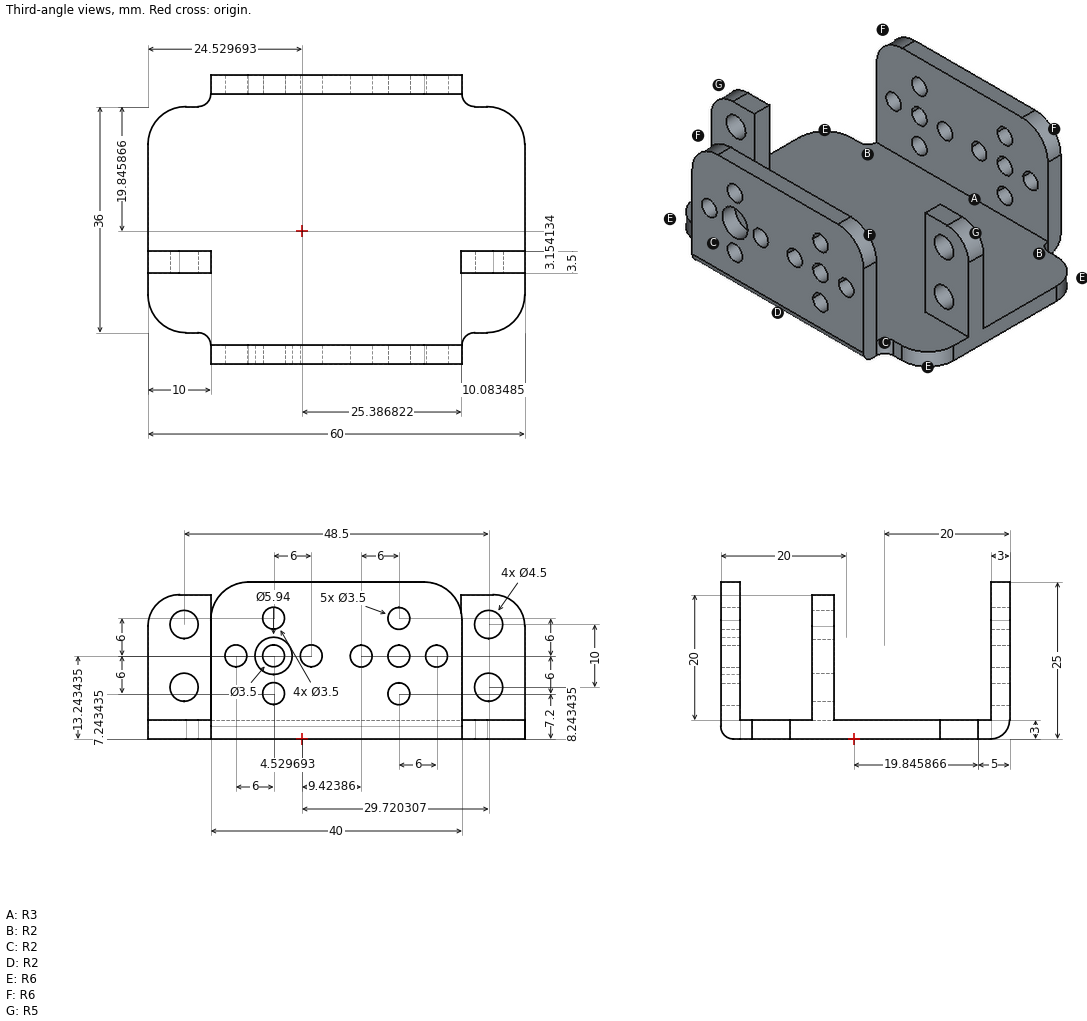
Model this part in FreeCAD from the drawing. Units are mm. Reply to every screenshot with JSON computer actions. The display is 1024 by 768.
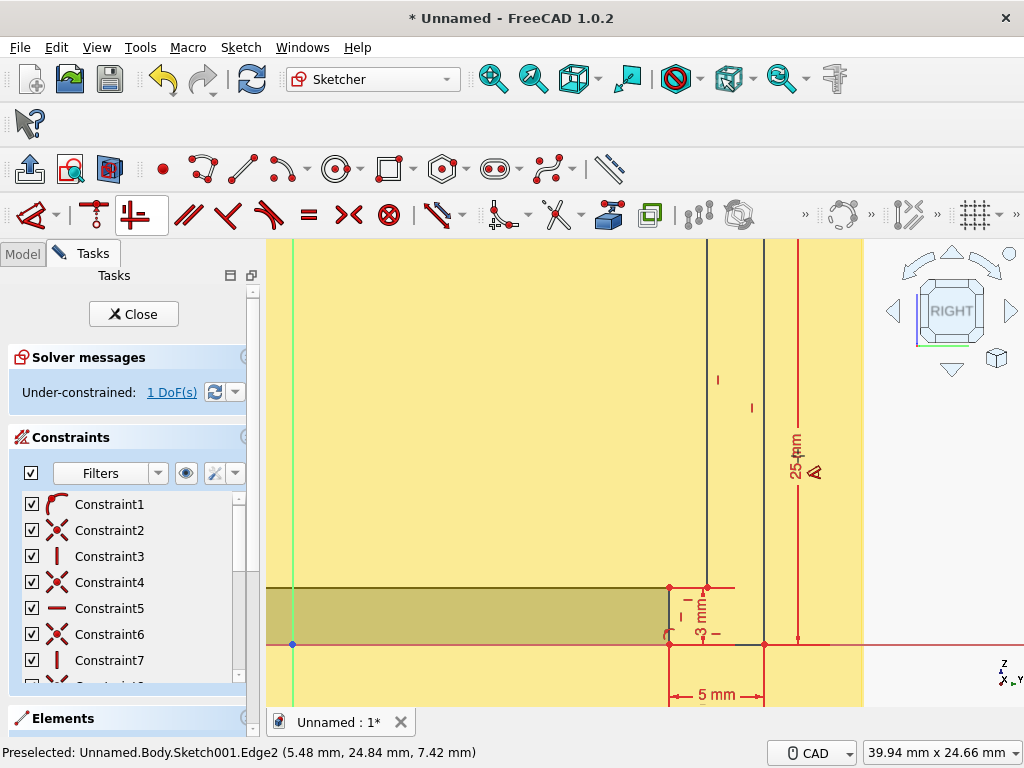
{"action": "left_click", "coordinate": [669, 645]}
{"action": "left_click", "coordinate": [482, 679]}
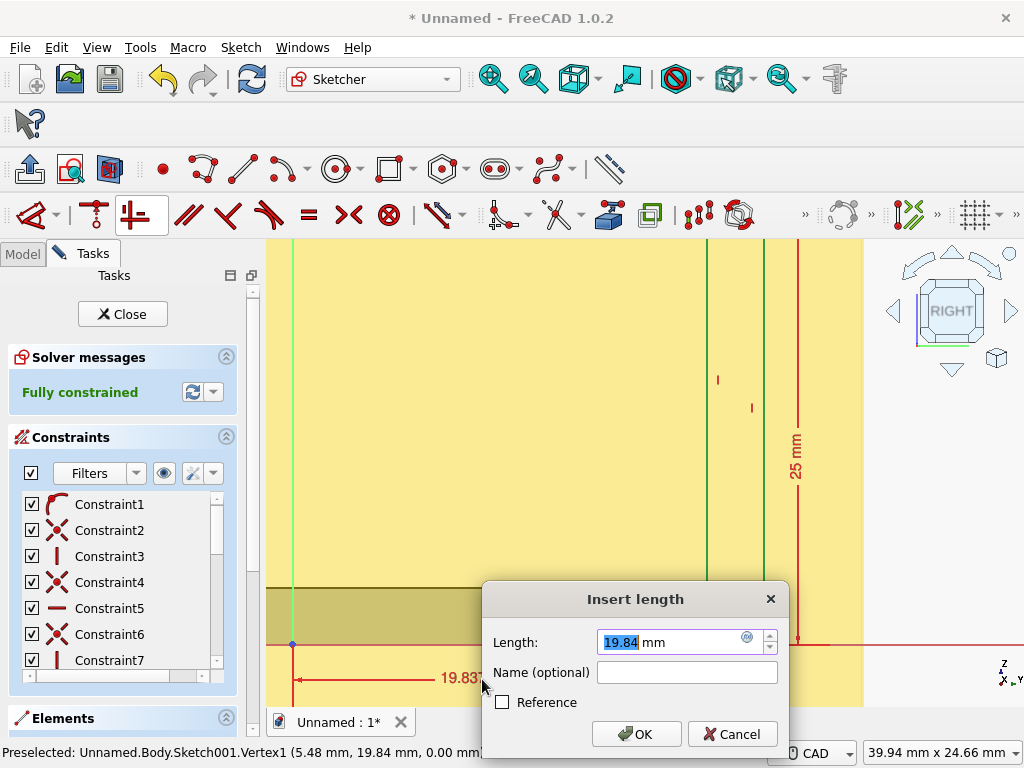
{"action": "type", "text": "19.845866"}
{"action": "key", "text": "Return"}
{"action": "key", "text": "Escape"}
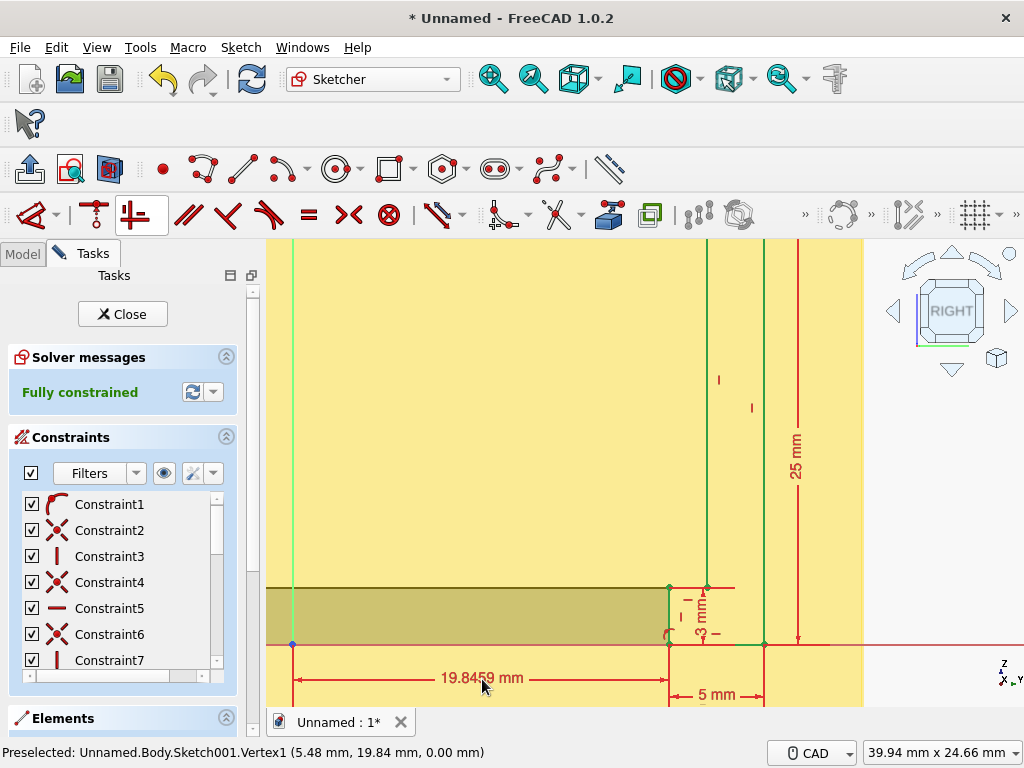
{"action": "left_click", "coordinate": [123, 314]}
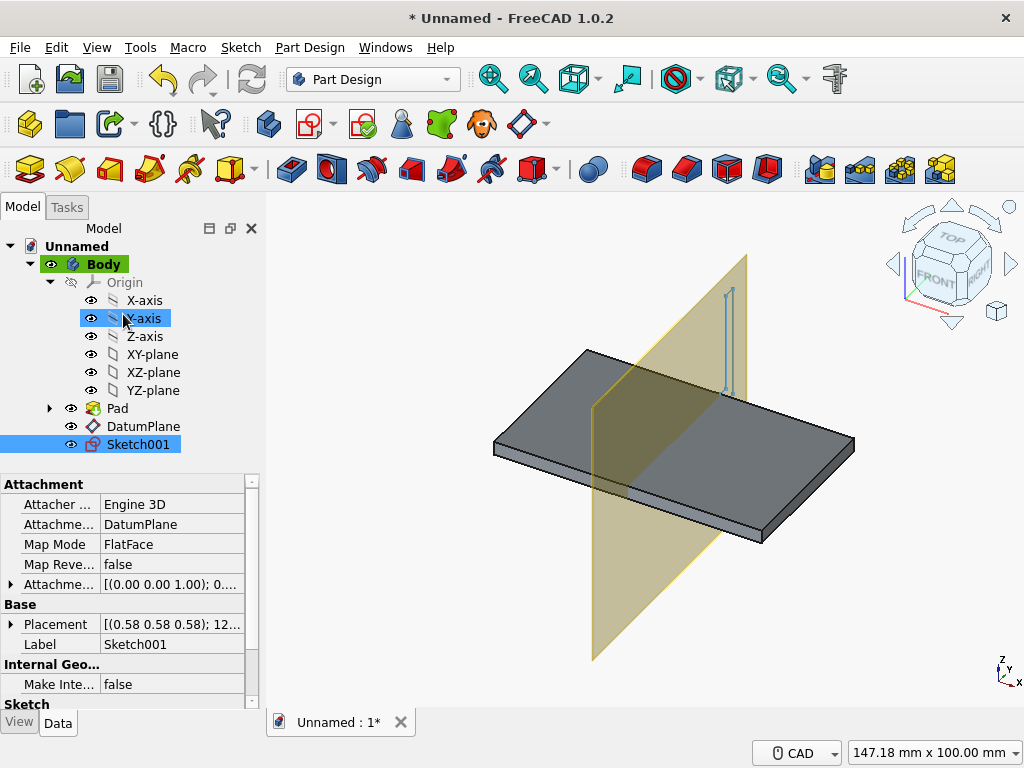
{"action": "left_click", "coordinate": [30, 170]}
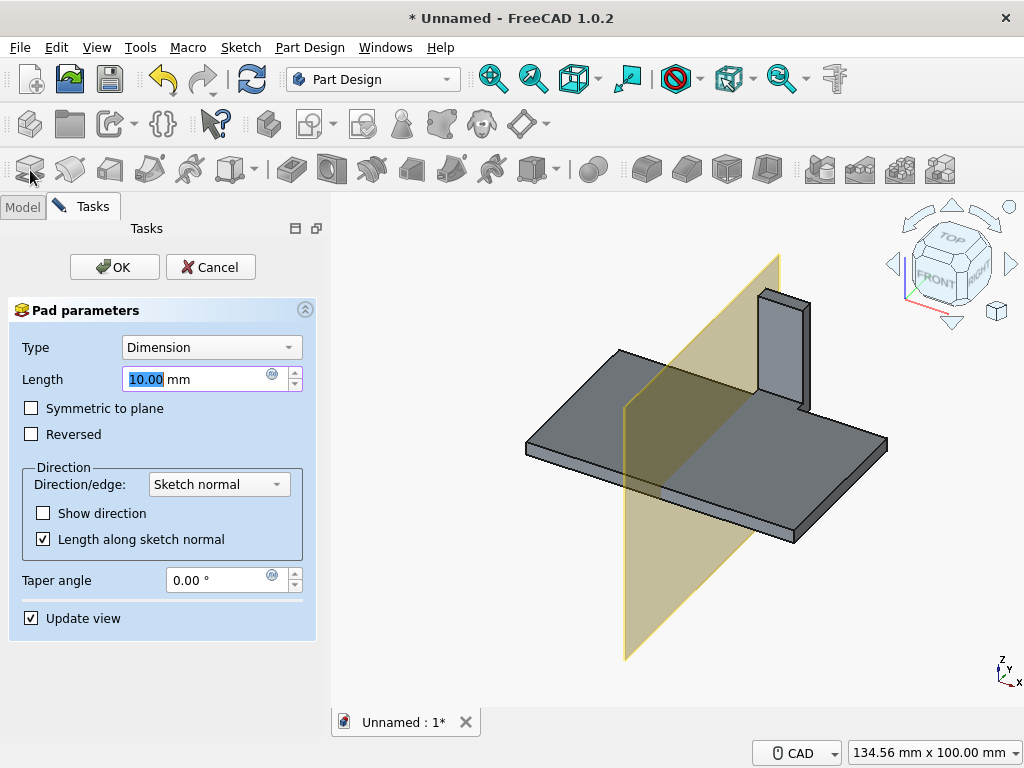
{"action": "type", "text": "40"}
{"action": "key", "text": "Tab"}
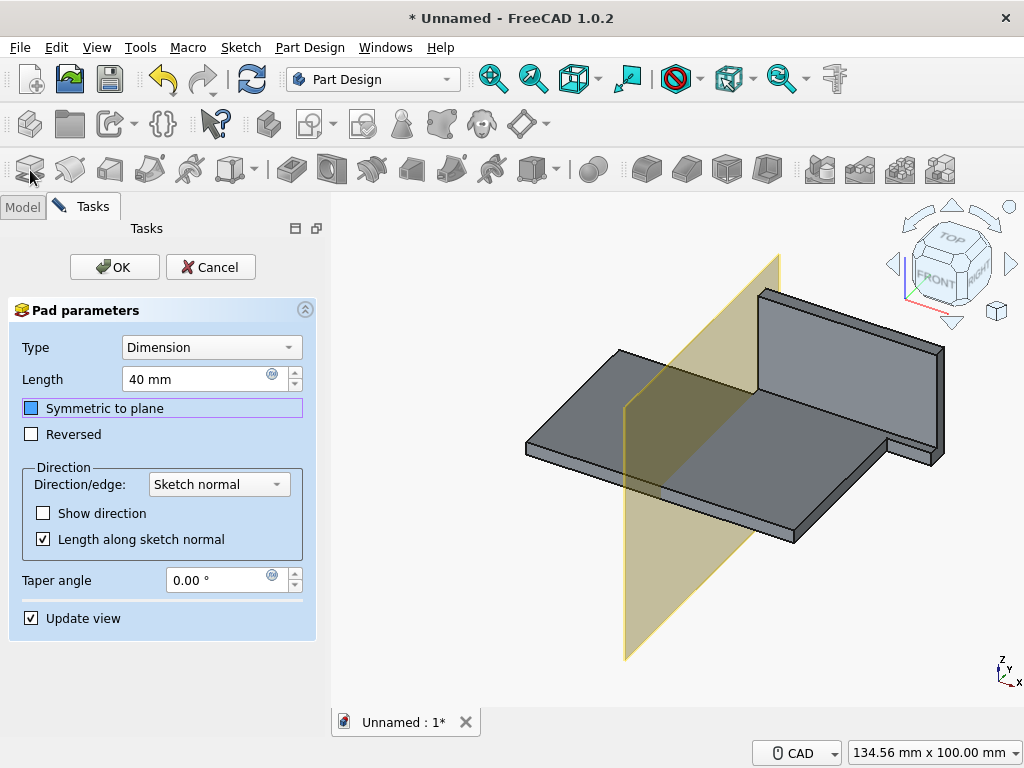
{"action": "left_click", "coordinate": [30, 408]}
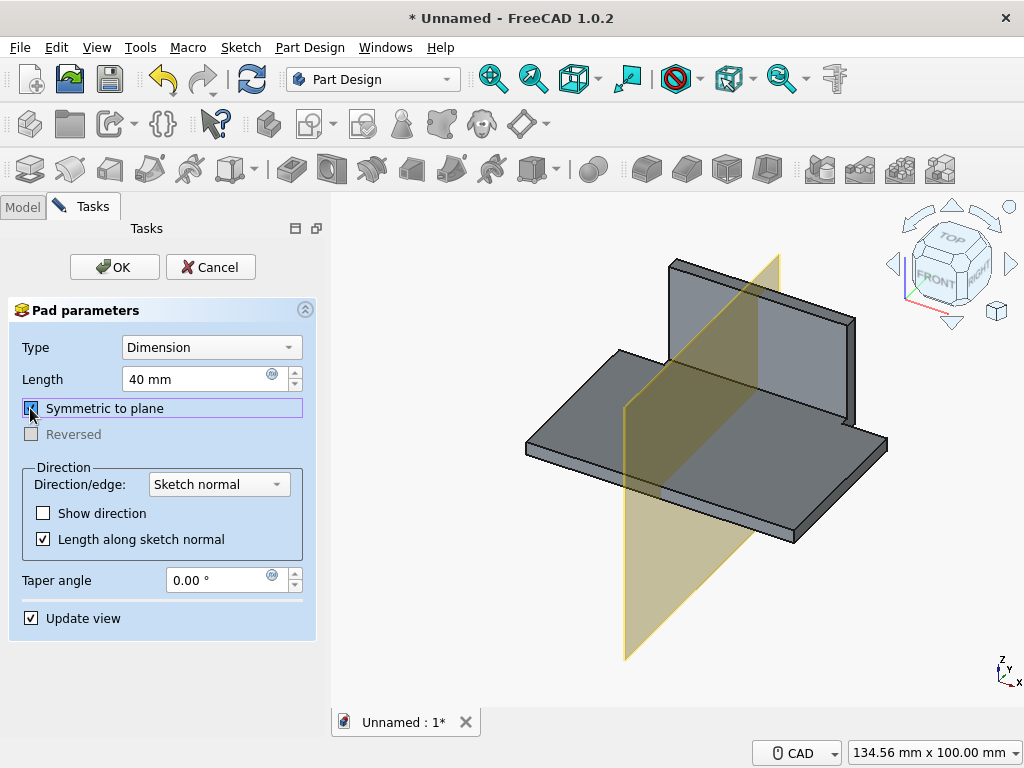
{"action": "left_click", "coordinate": [115, 267]}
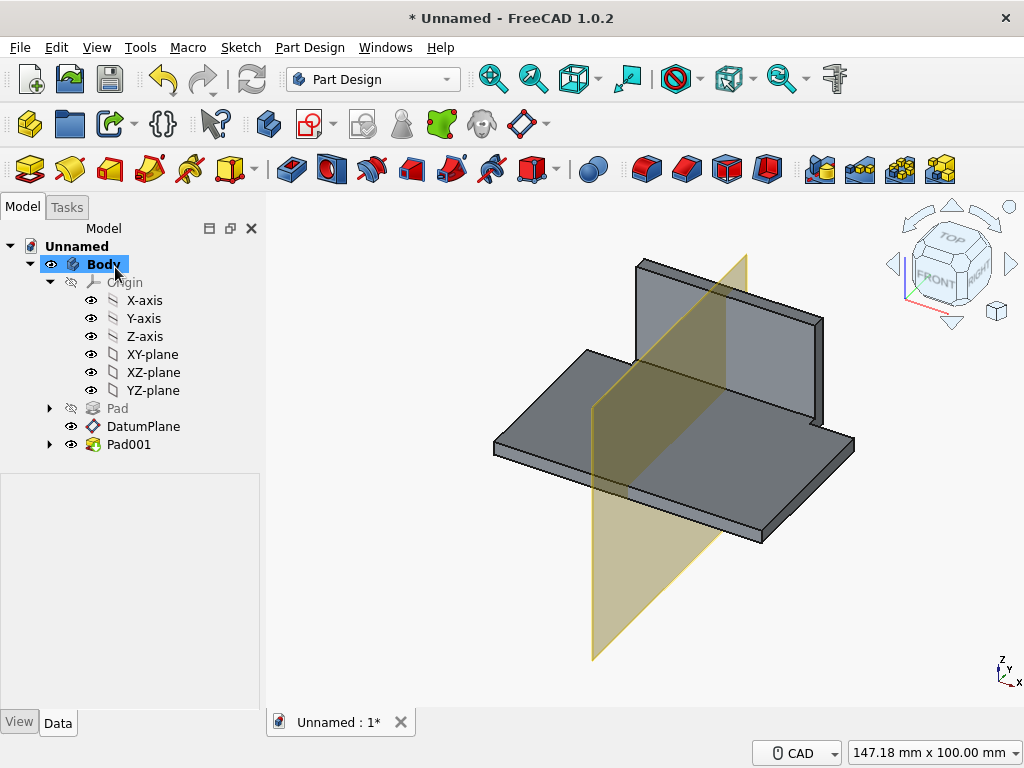
{"action": "left_click", "coordinate": [116, 426]}
{"action": "key", "text": "space"}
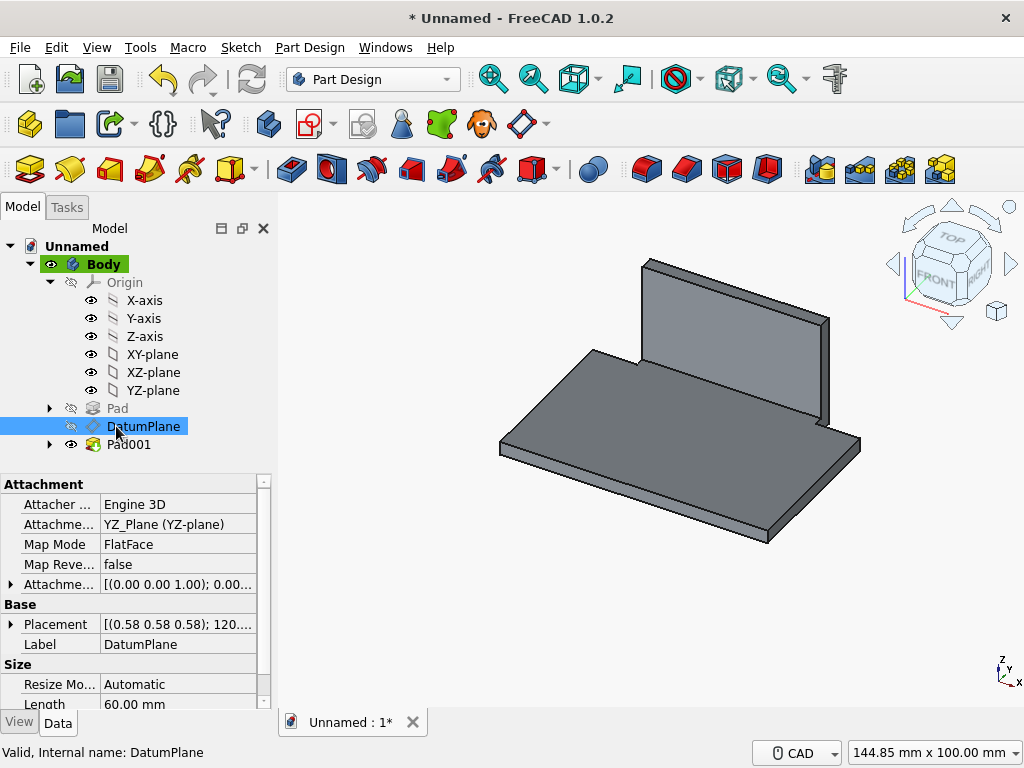
{"action": "key", "text": "0"}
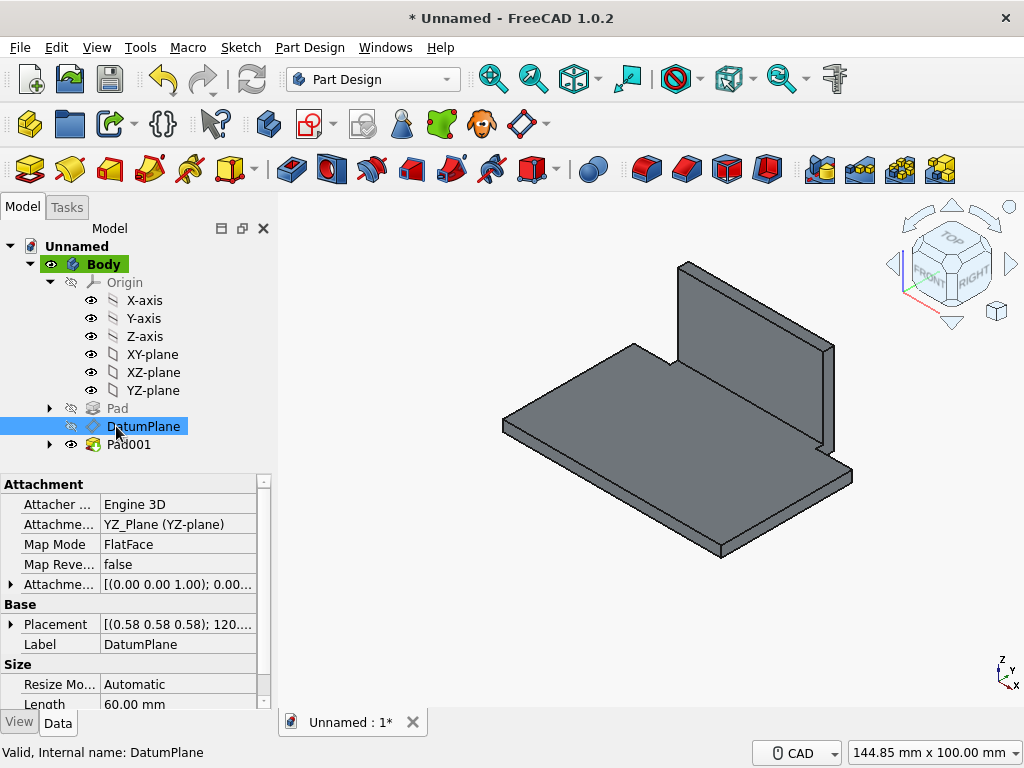
{"action": "key", "text": "2"}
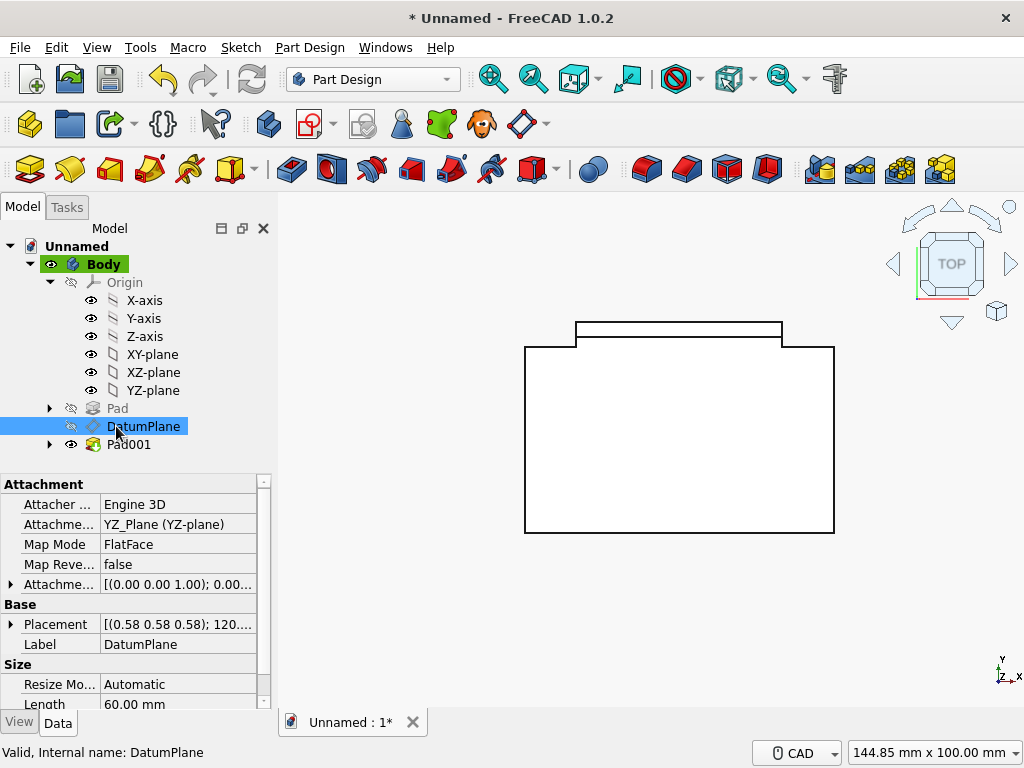
{"action": "left_click", "coordinate": [494, 80]}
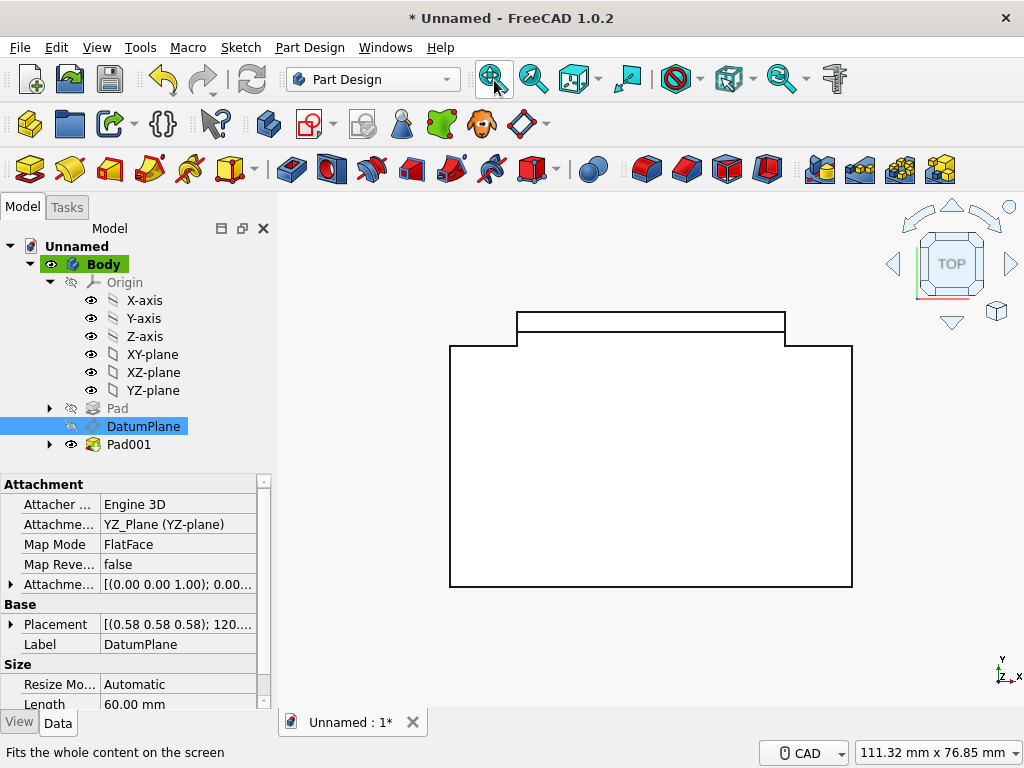
{"action": "key", "text": "1"}